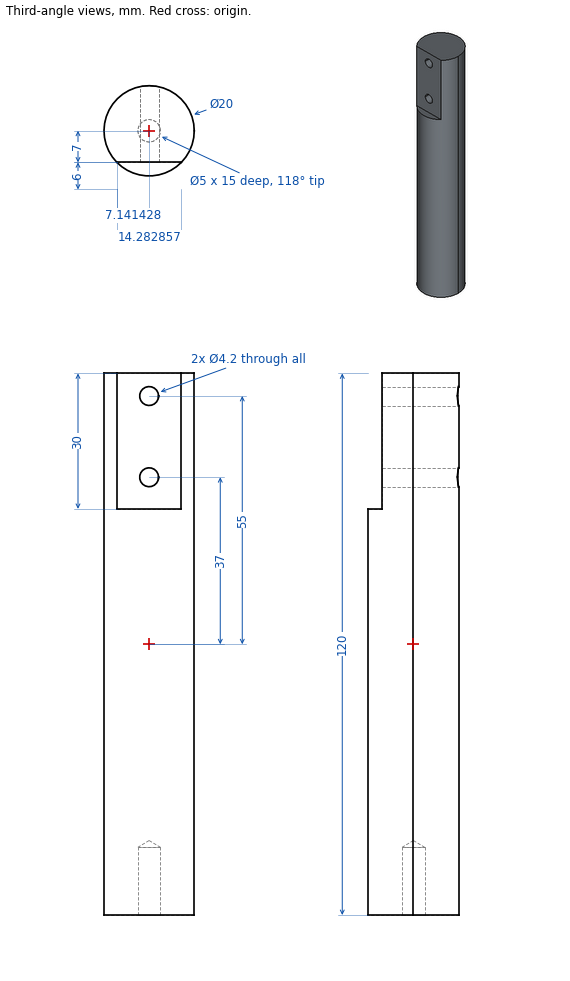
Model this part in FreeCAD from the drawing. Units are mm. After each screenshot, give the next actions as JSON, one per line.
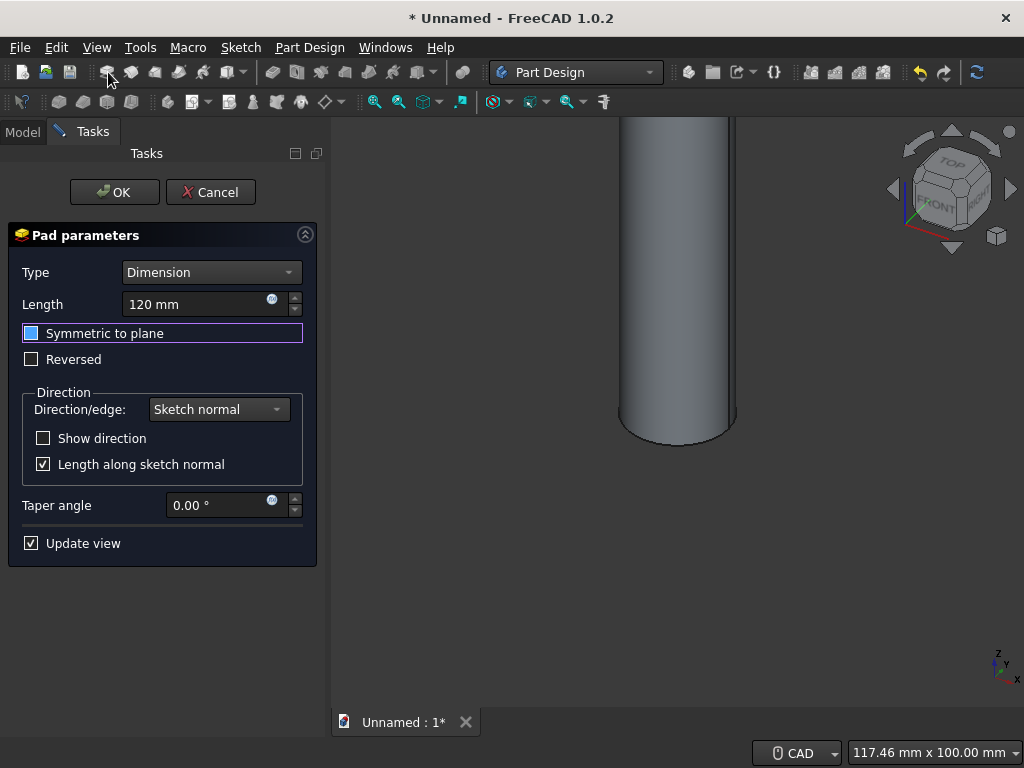
{"action": "left_click", "coordinate": [30, 333]}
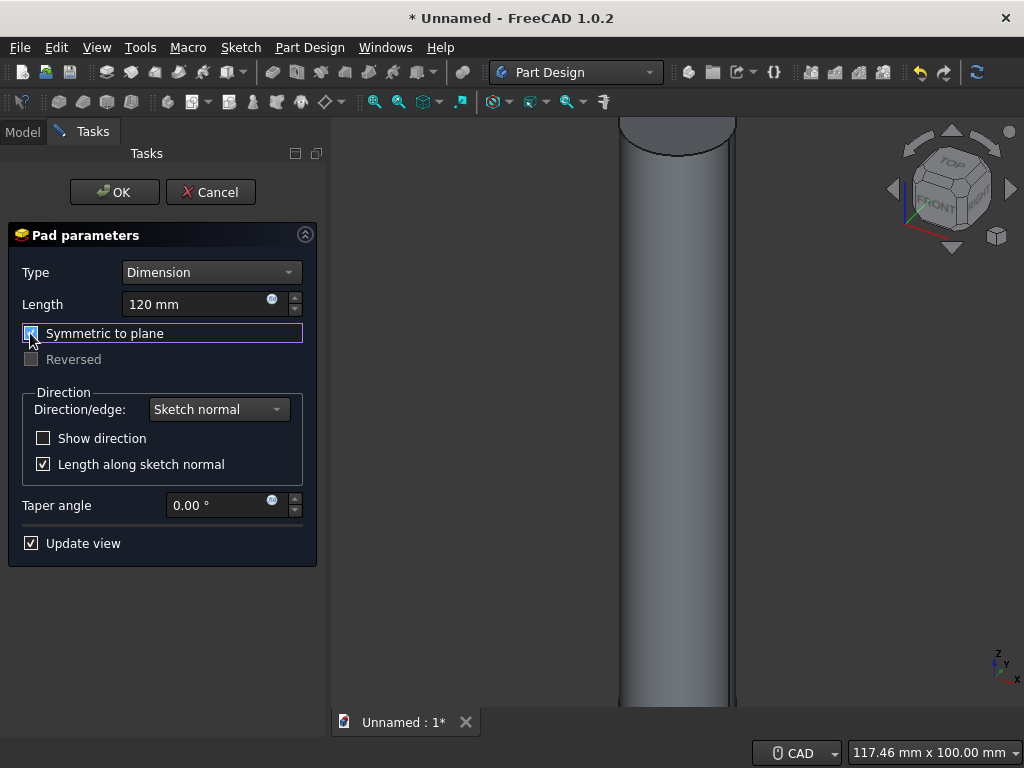
{"action": "left_click", "coordinate": [115, 192]}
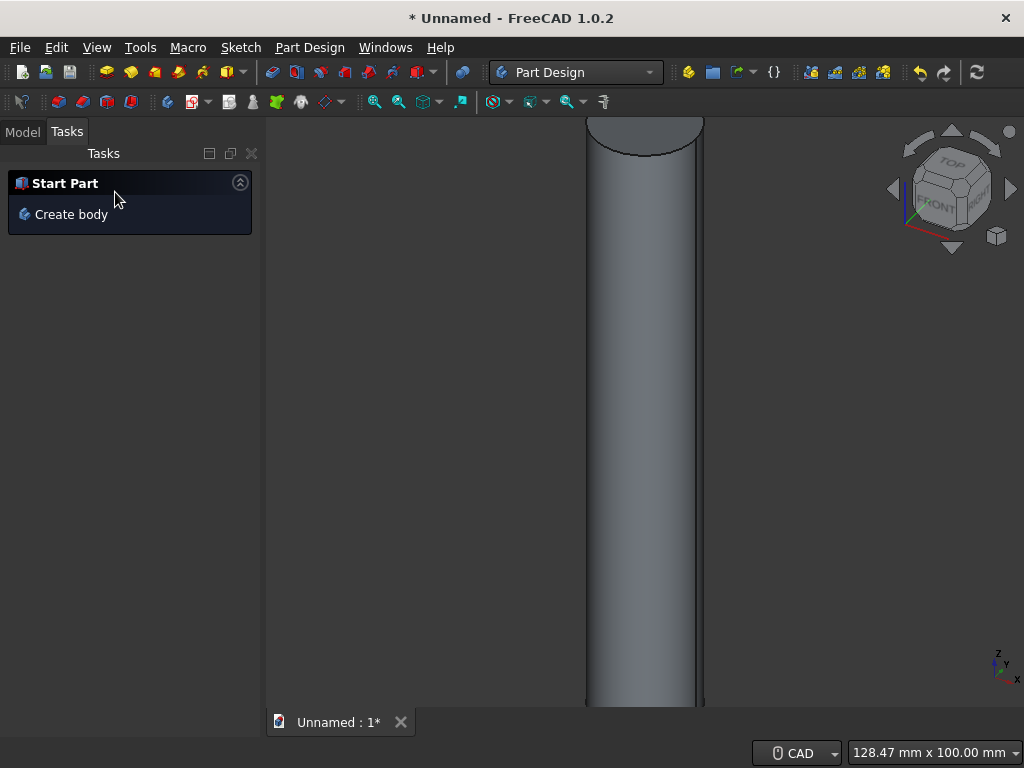
{"action": "left_click", "coordinate": [376, 102]}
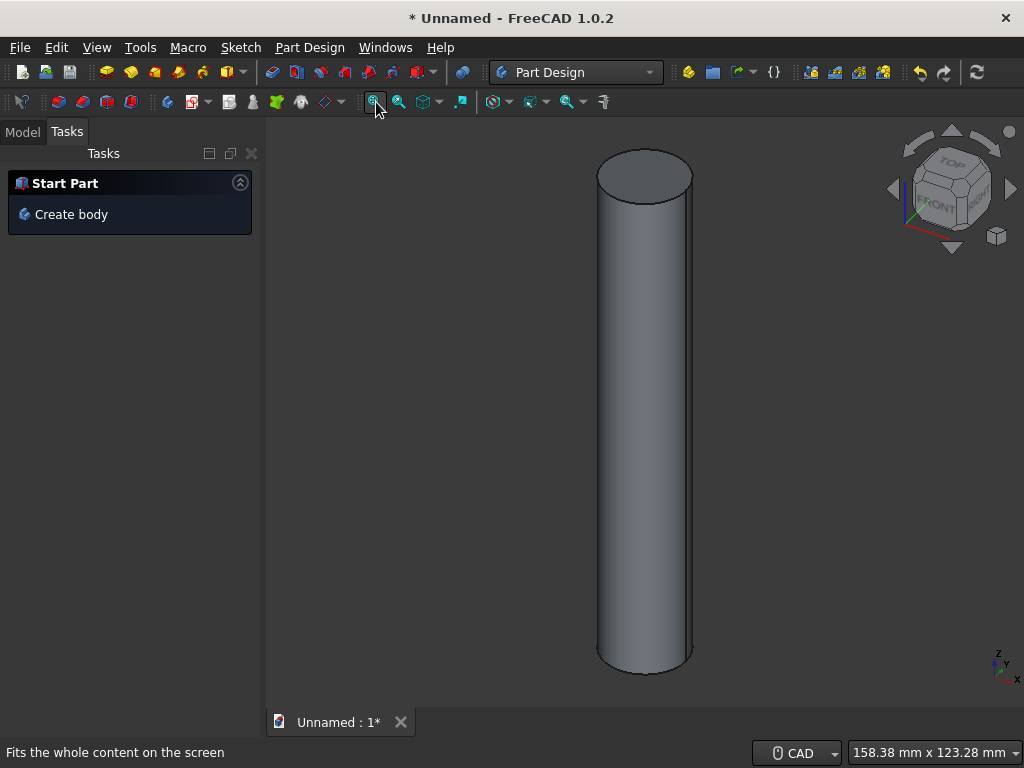
{"action": "key", "text": "5"}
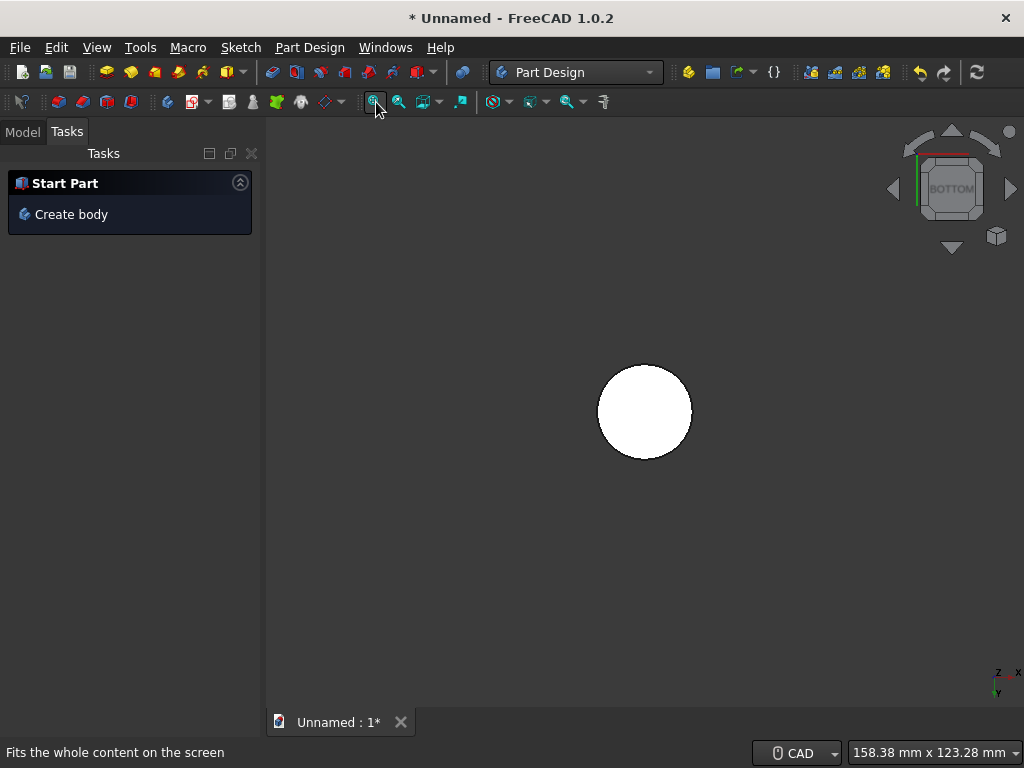
{"action": "left_click", "coordinate": [376, 102]}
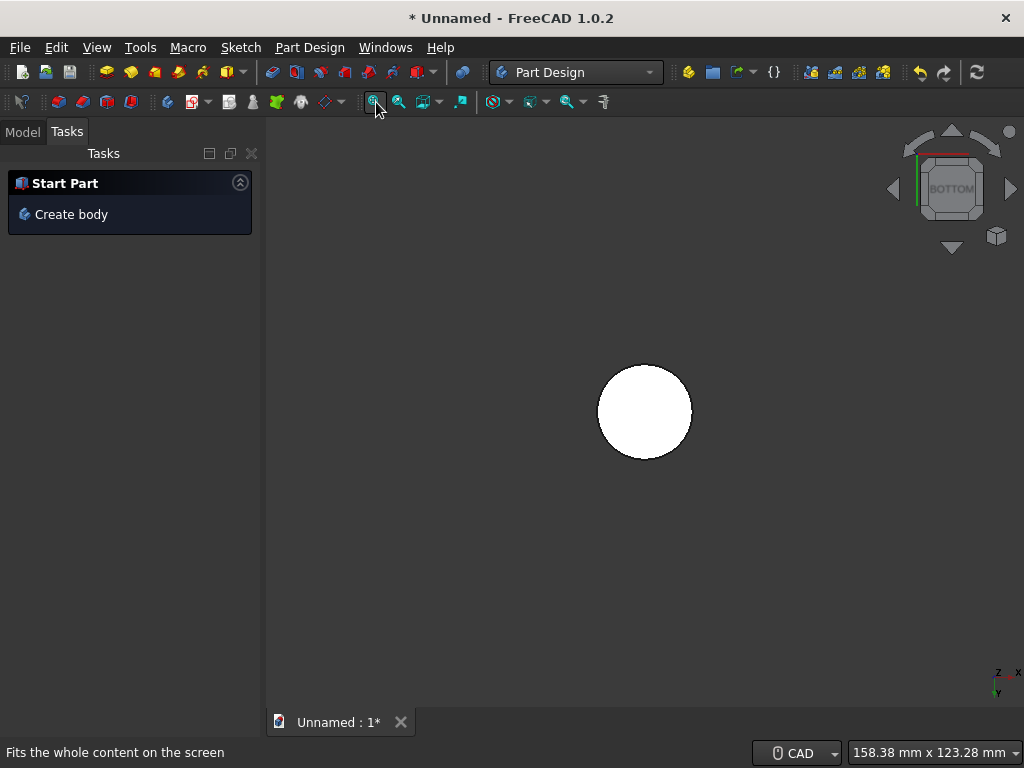
{"action": "left_click", "coordinate": [645, 411]}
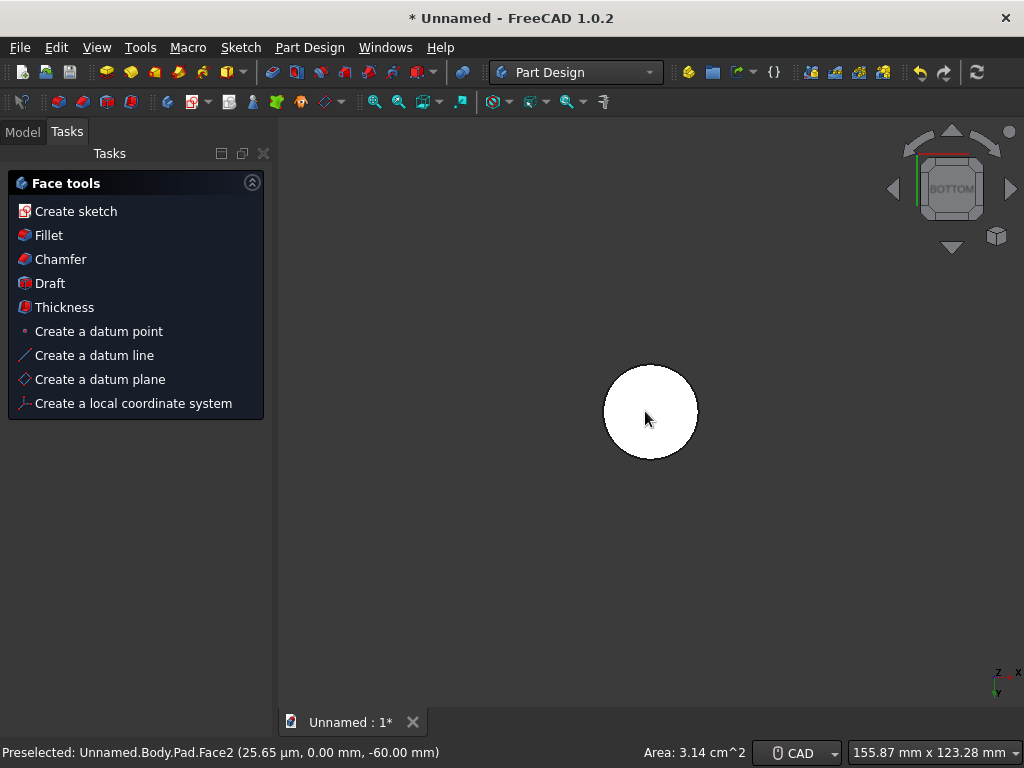
{"action": "left_click", "coordinate": [192, 102]}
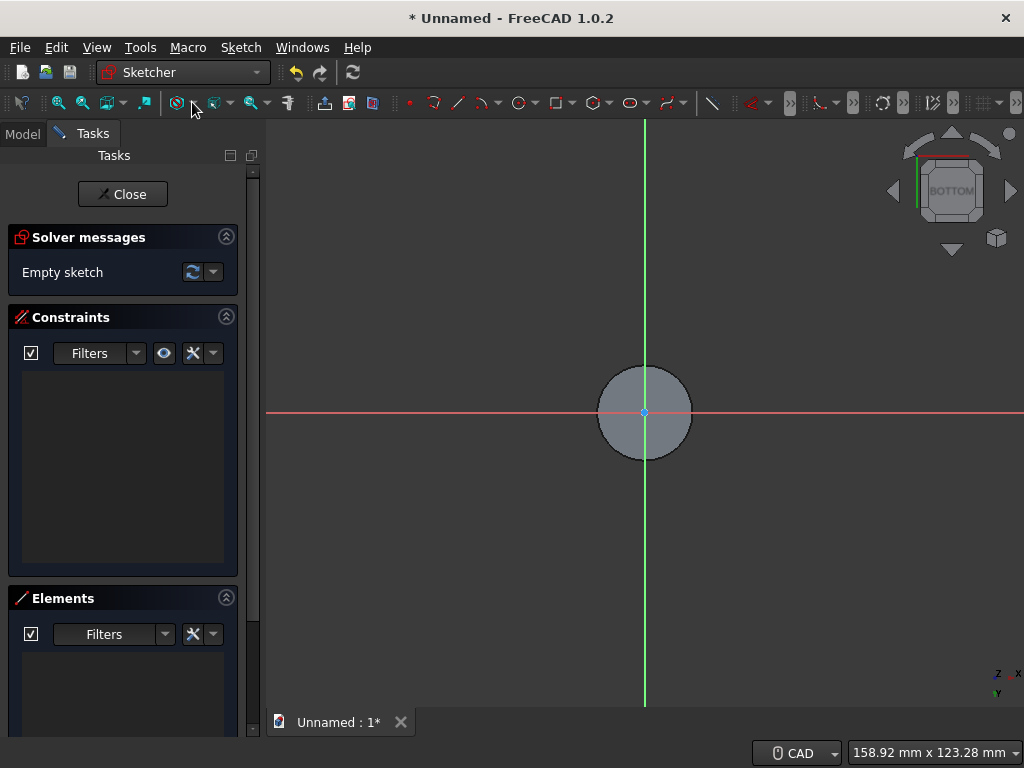
{"action": "scroll", "coordinate": [649, 413], "scroll_direction": "up", "scroll_amount": 14}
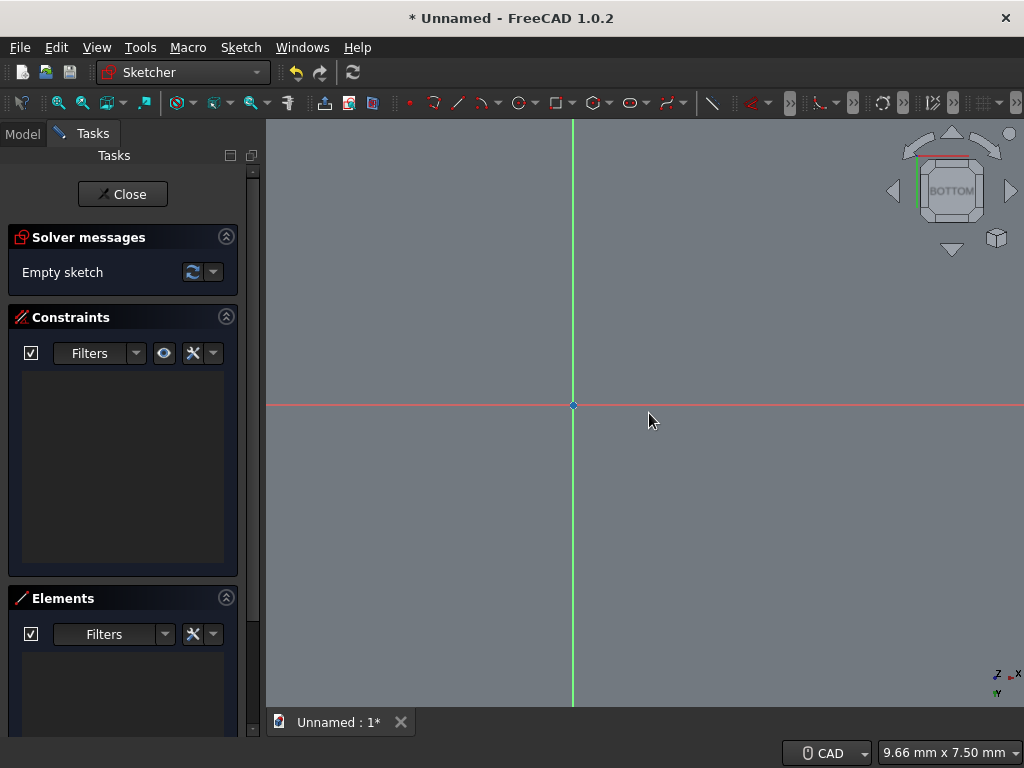
{"action": "left_click", "coordinate": [520, 104]}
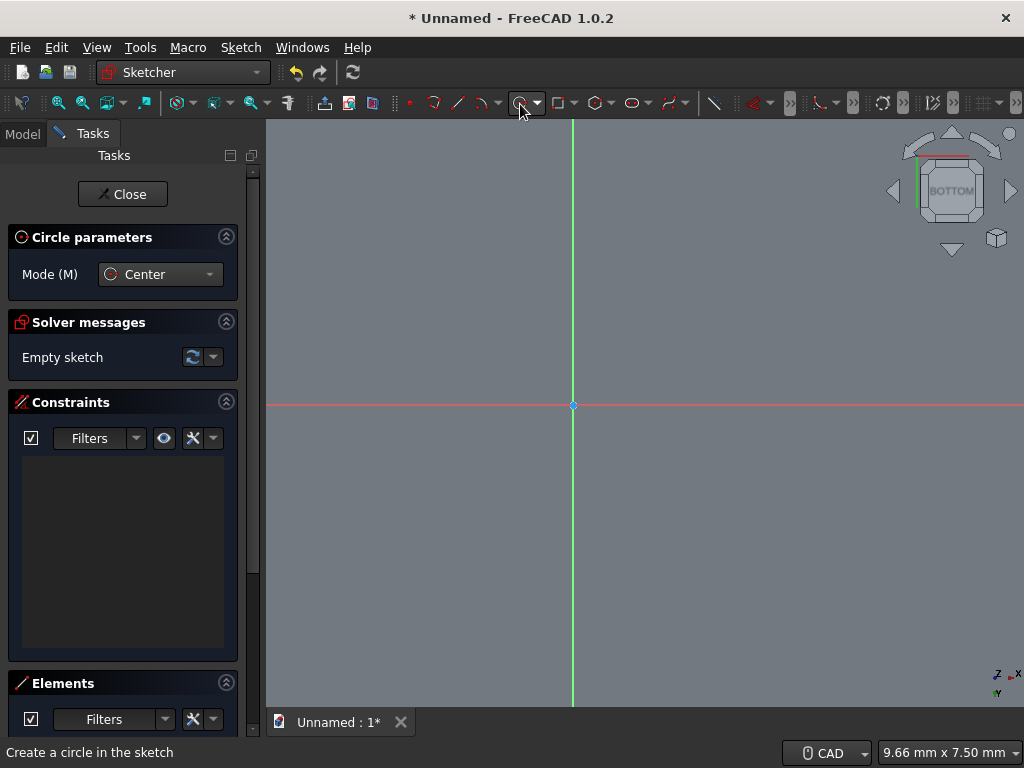
{"action": "left_click", "coordinate": [573, 405]}
{"action": "left_click", "coordinate": [712, 267]}
{"action": "key", "text": "Escape"}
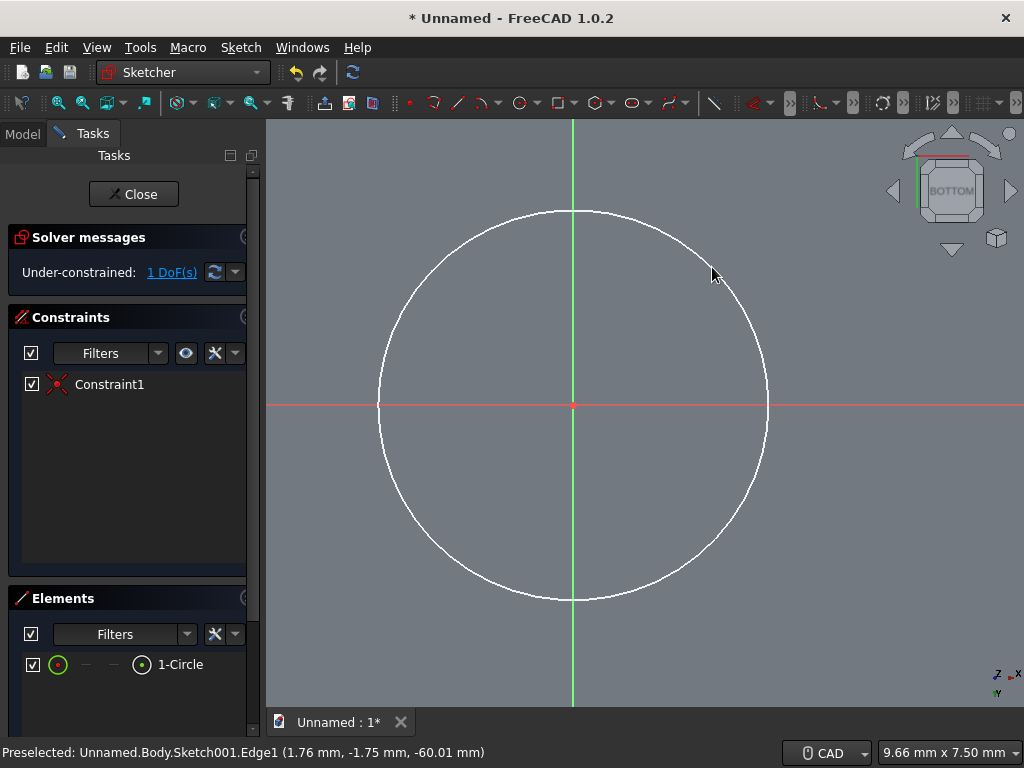
{"action": "left_click", "coordinate": [754, 104]}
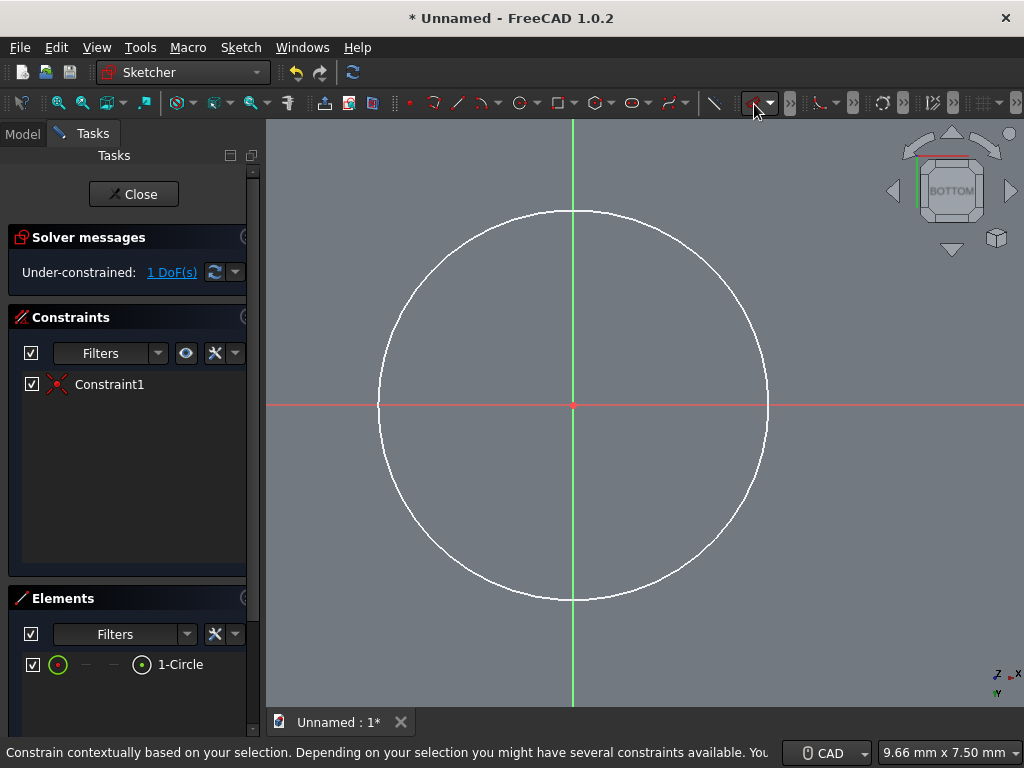
{"action": "left_click", "coordinate": [711, 267]}
{"action": "left_click", "coordinate": [734, 244]}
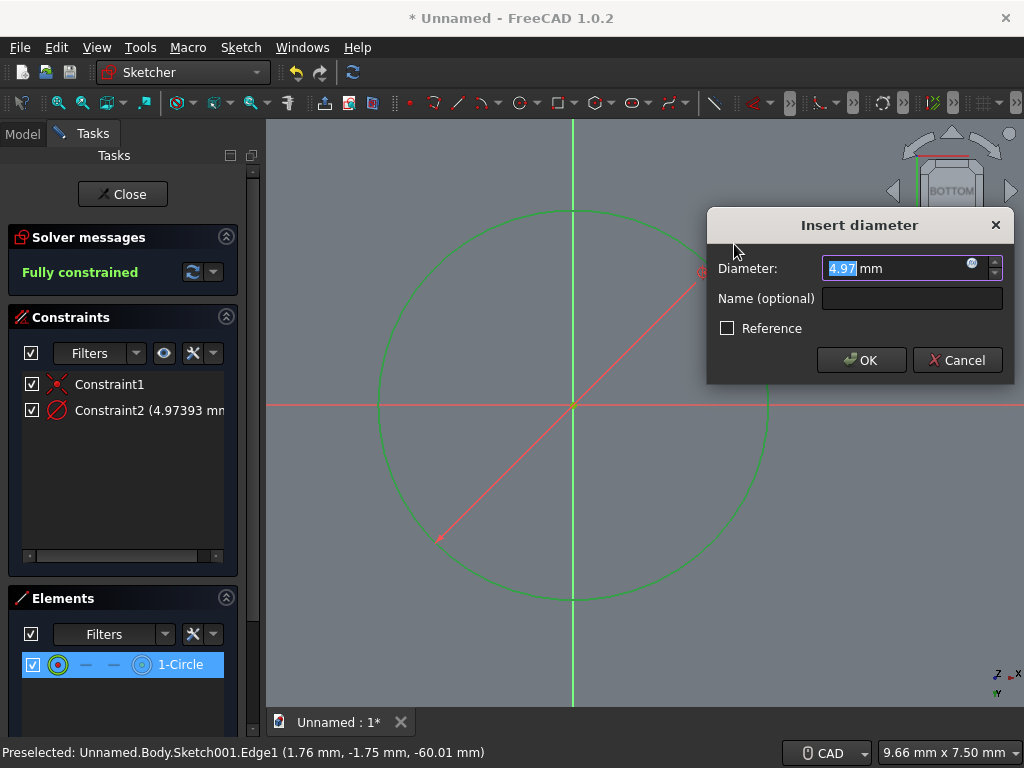
{"action": "type", "text": "5"}
{"action": "key", "text": "Return"}
{"action": "key", "text": "Escape"}